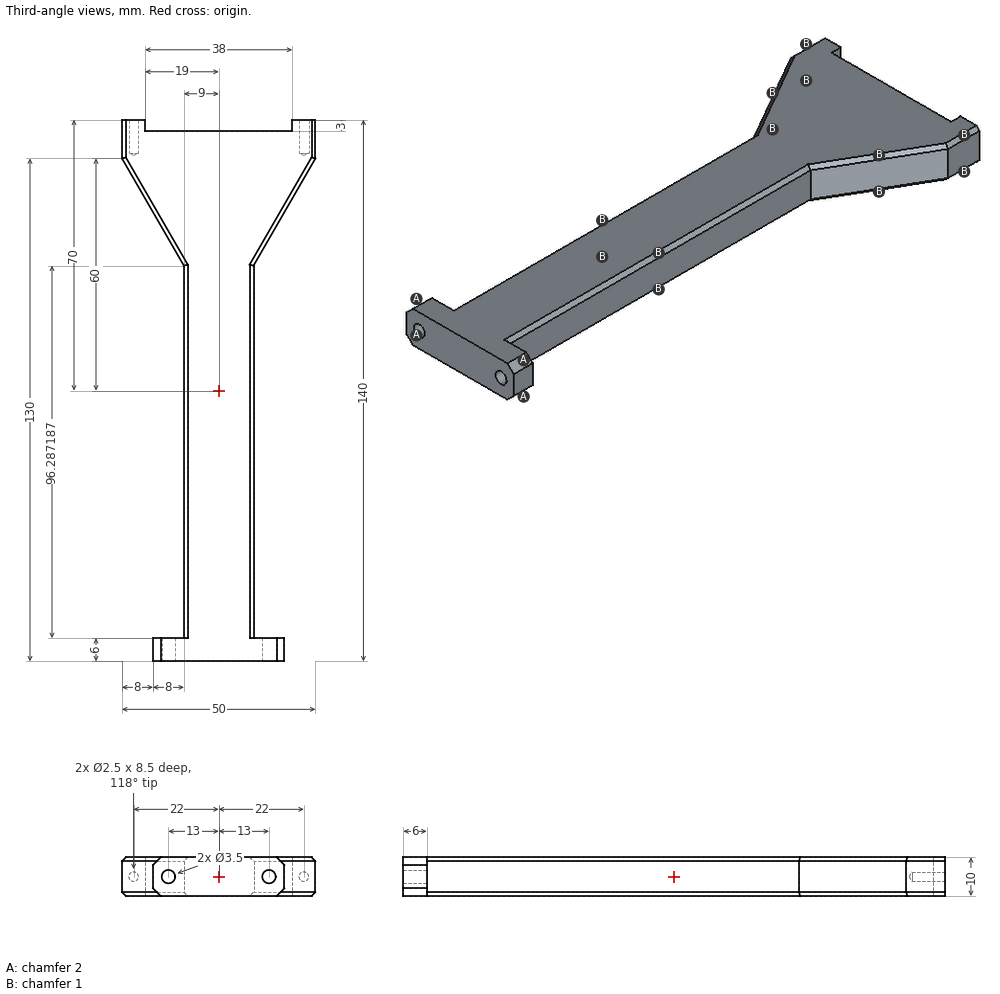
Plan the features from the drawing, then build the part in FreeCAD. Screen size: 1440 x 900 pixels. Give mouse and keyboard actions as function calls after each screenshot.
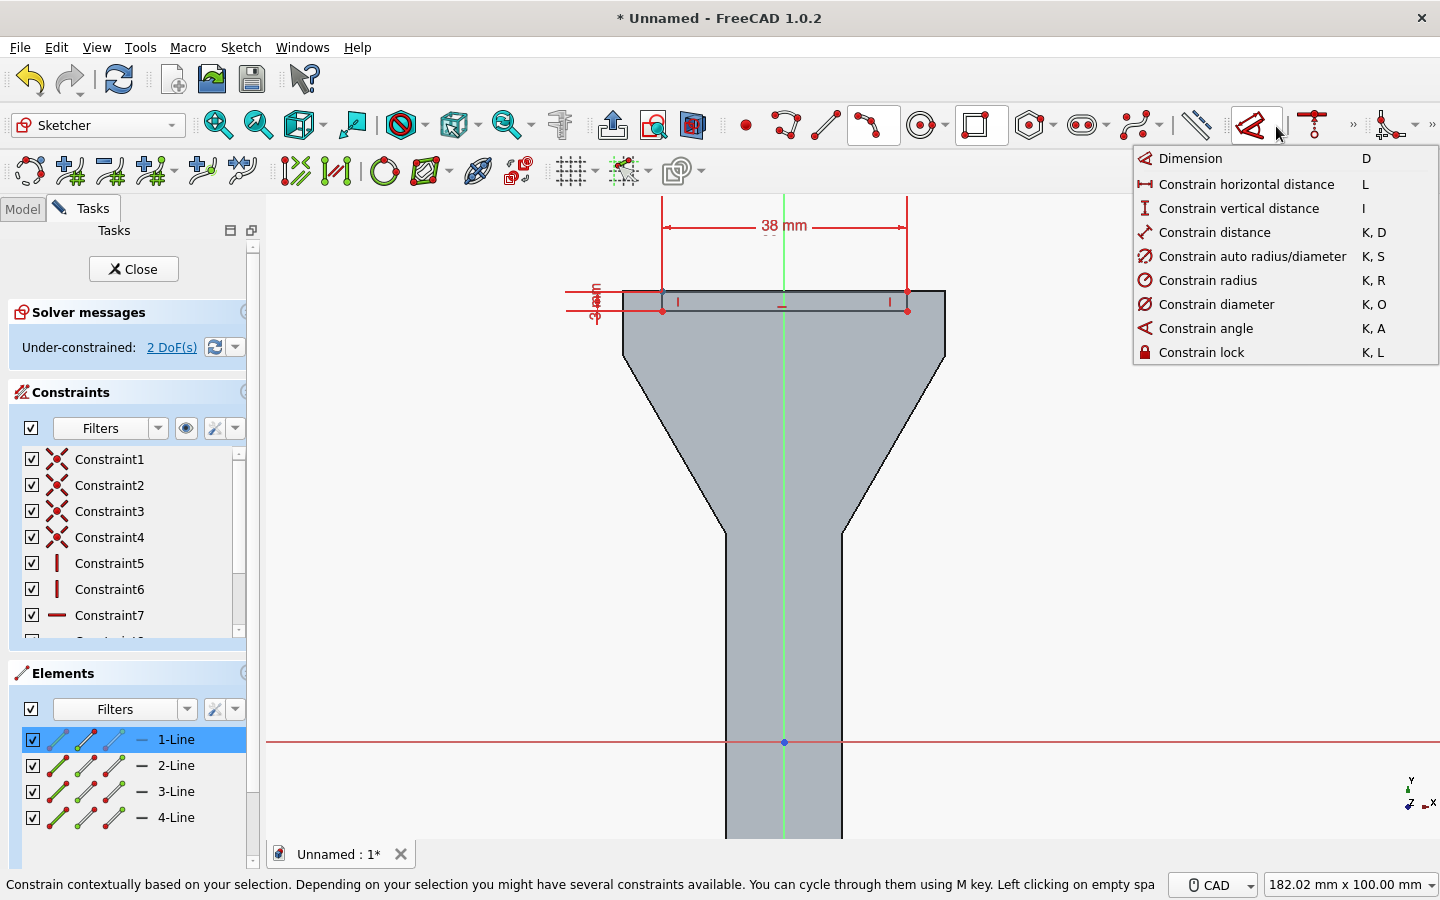
click(1286, 184)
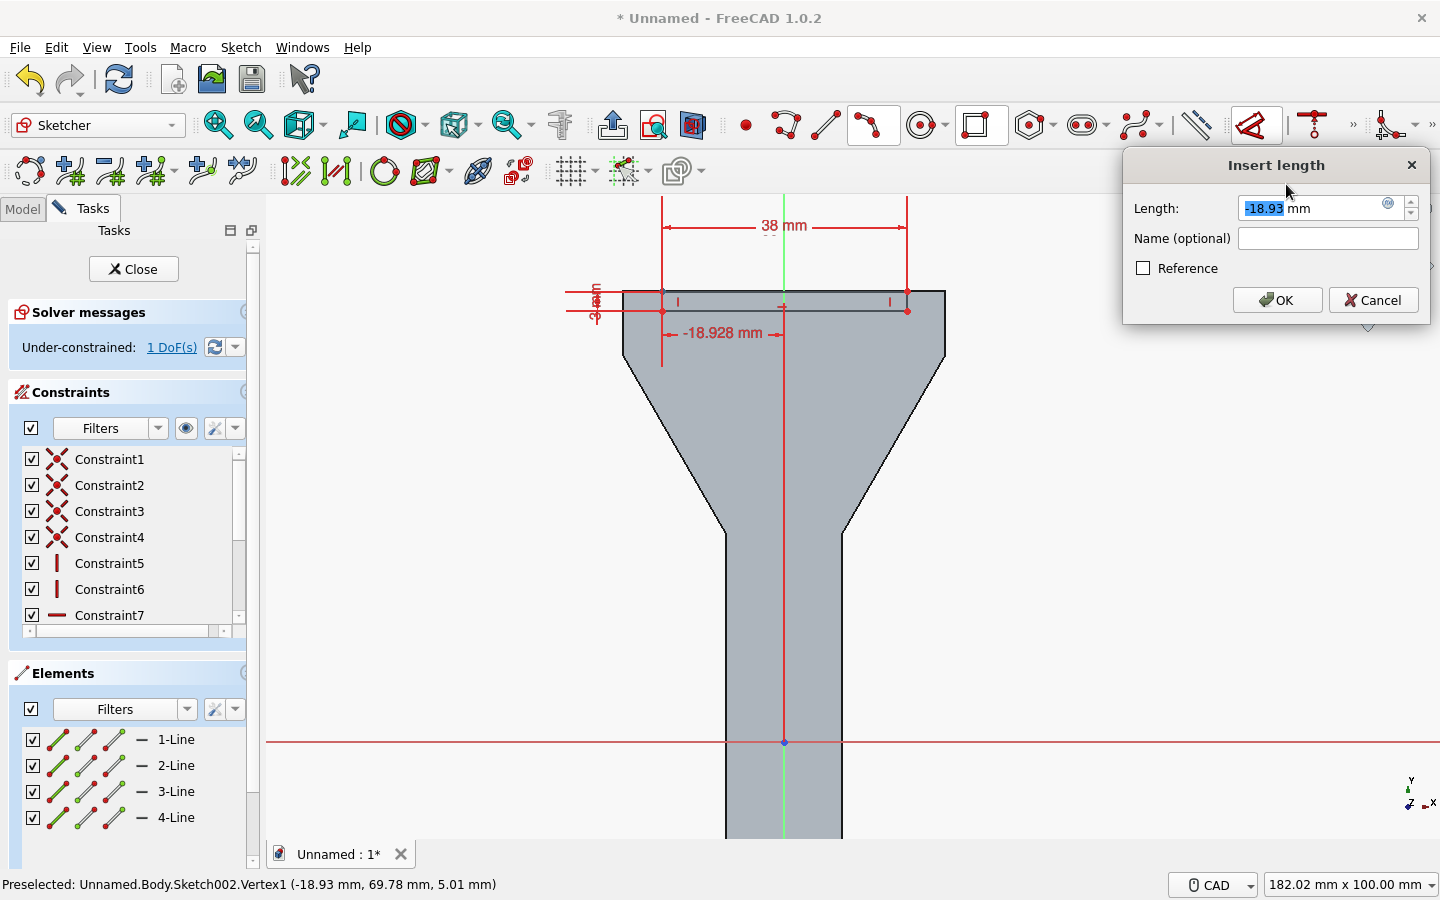
text(-19)
key(Return)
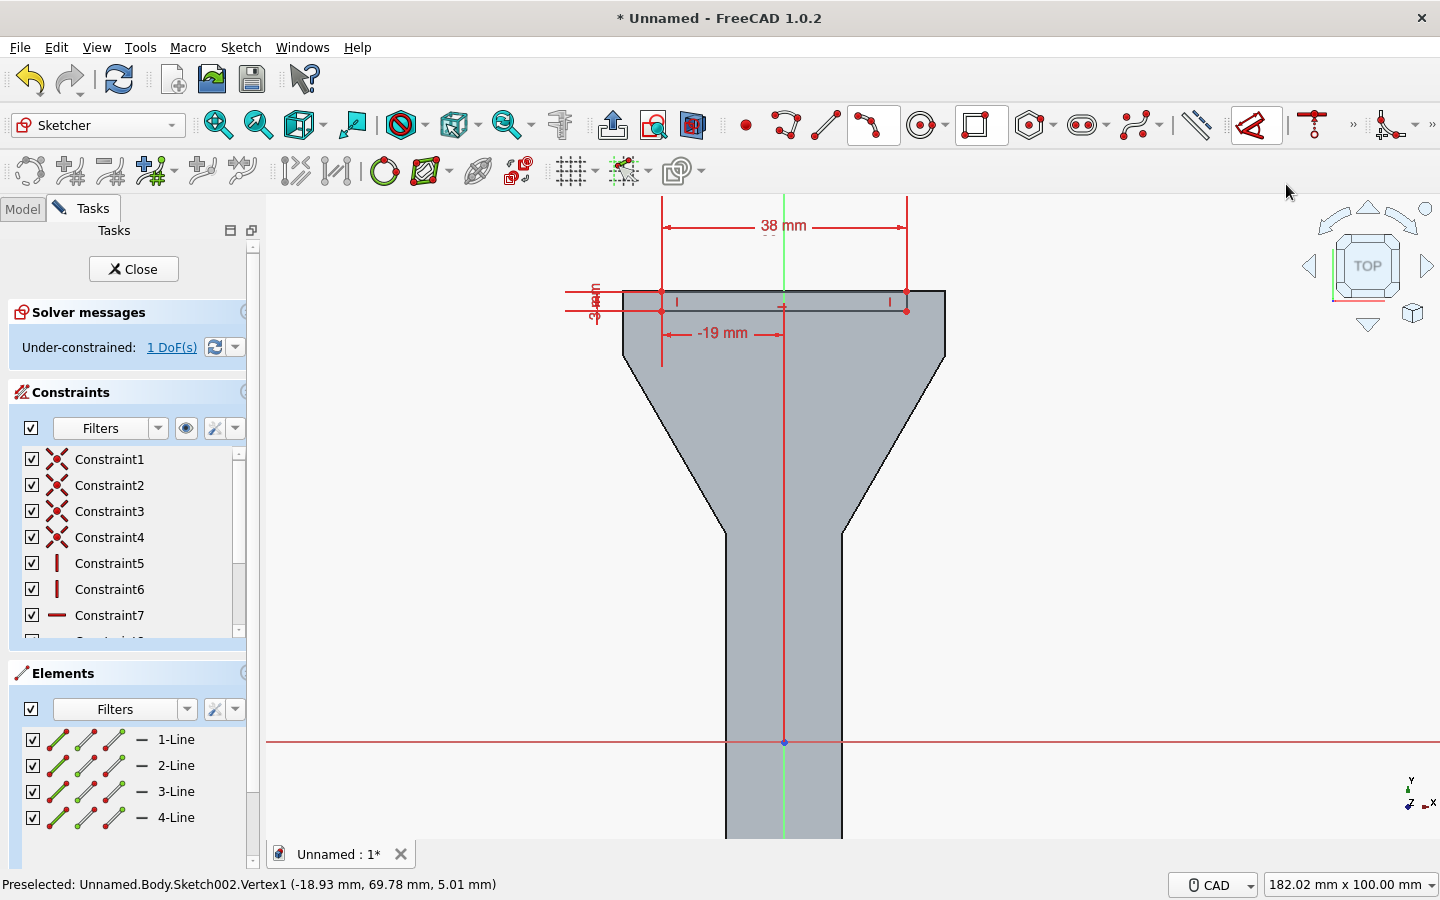
click(662, 292)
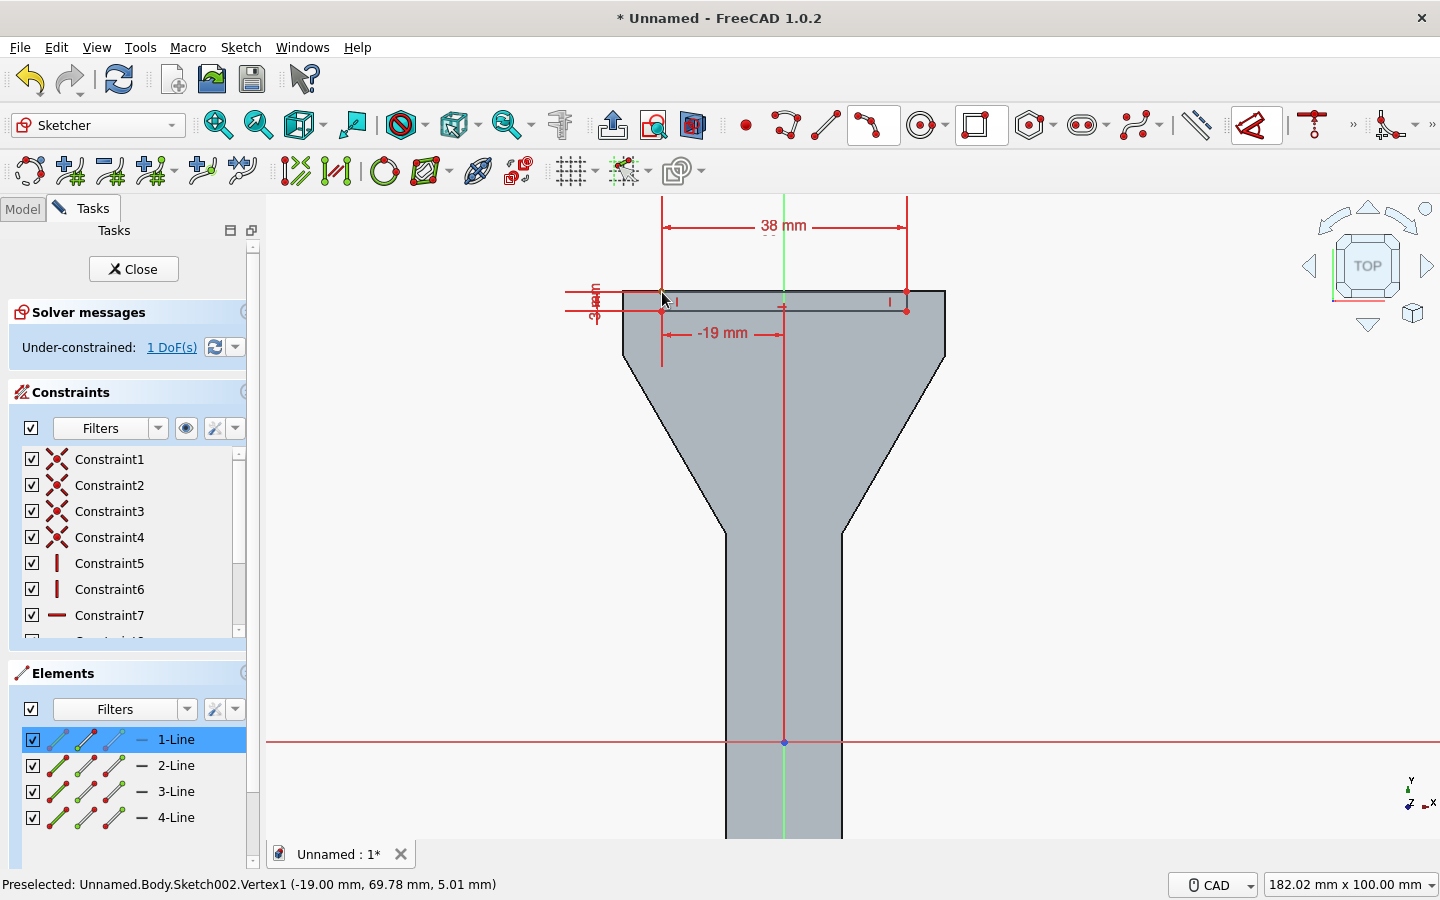
click(1276, 126)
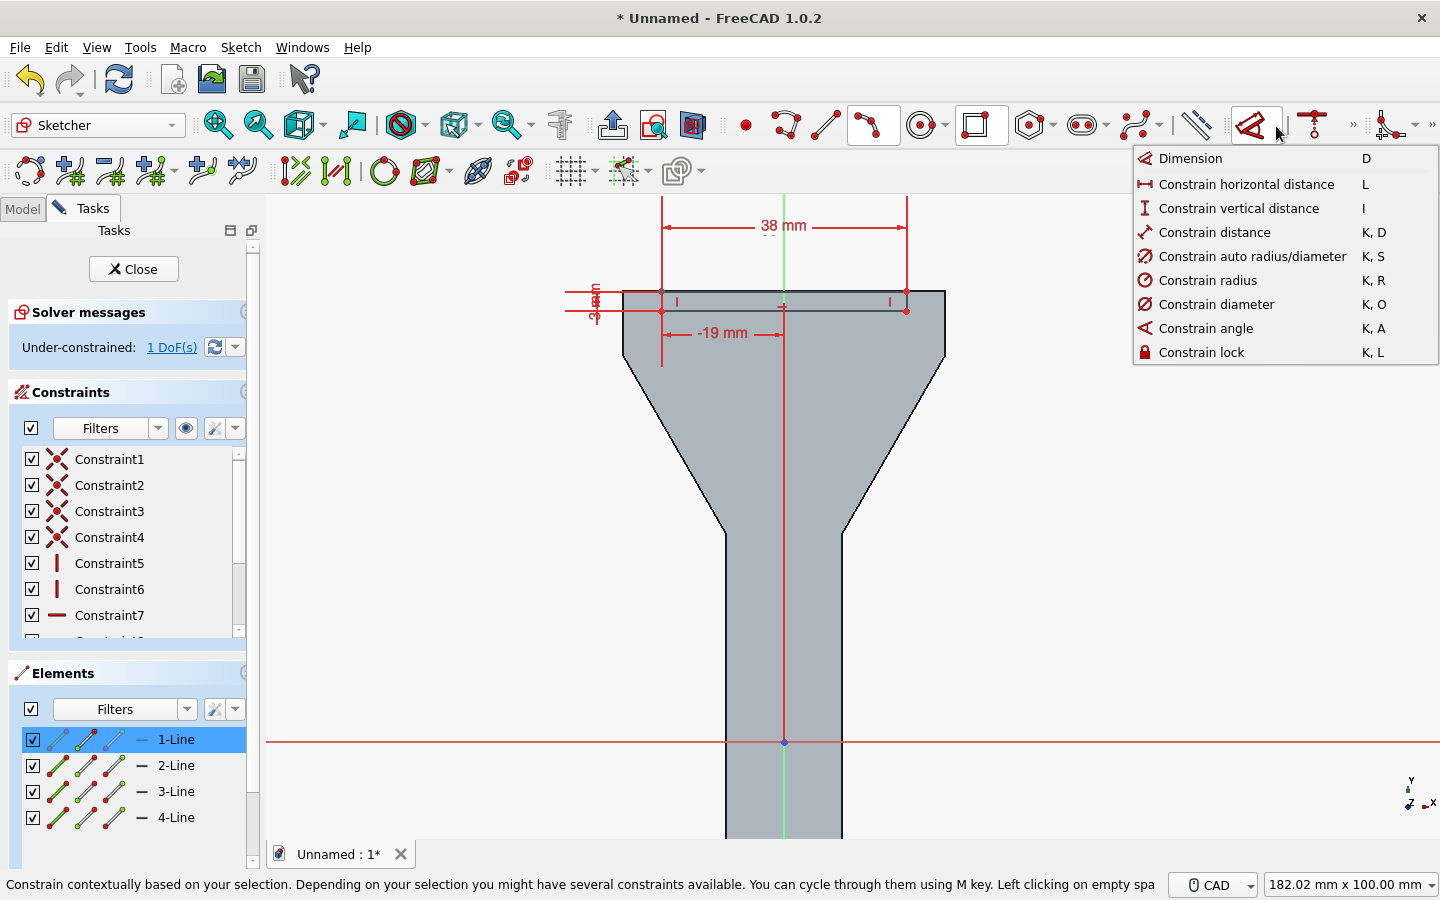
click(1286, 208)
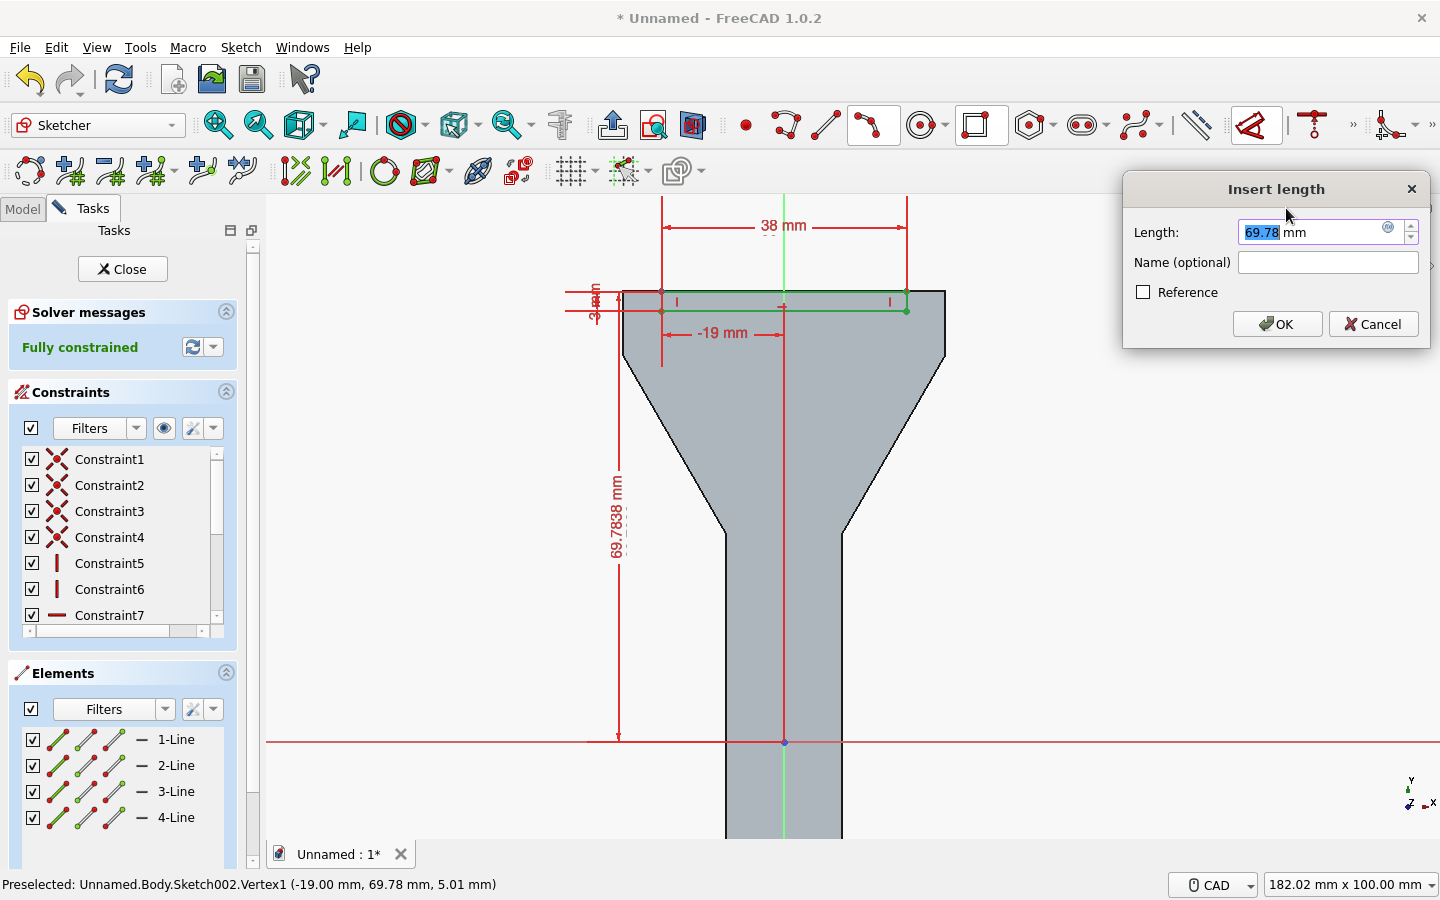
text(70)
key(Return)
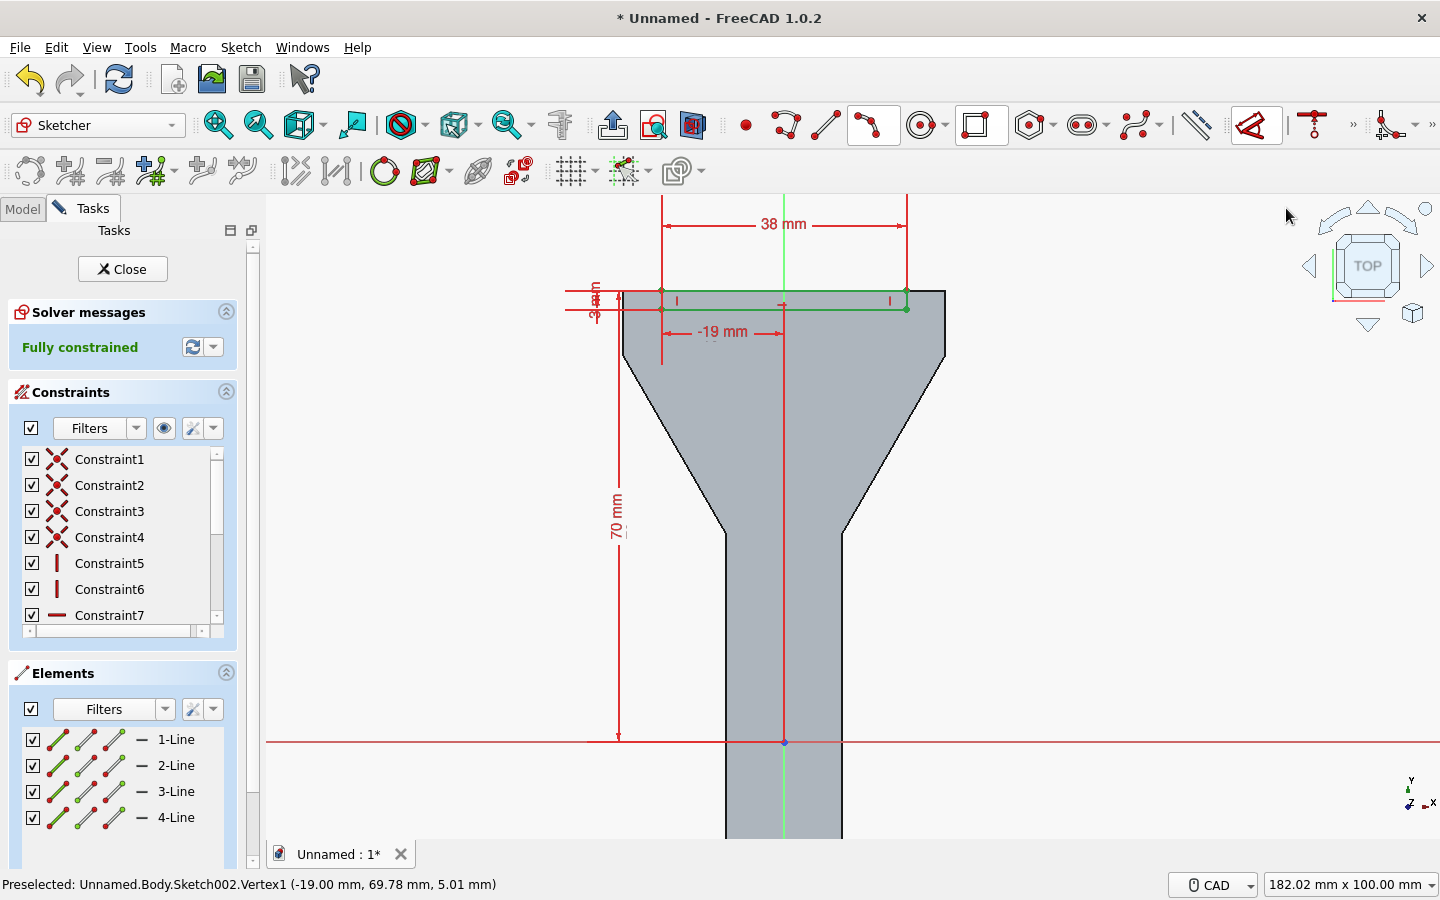
click(123, 269)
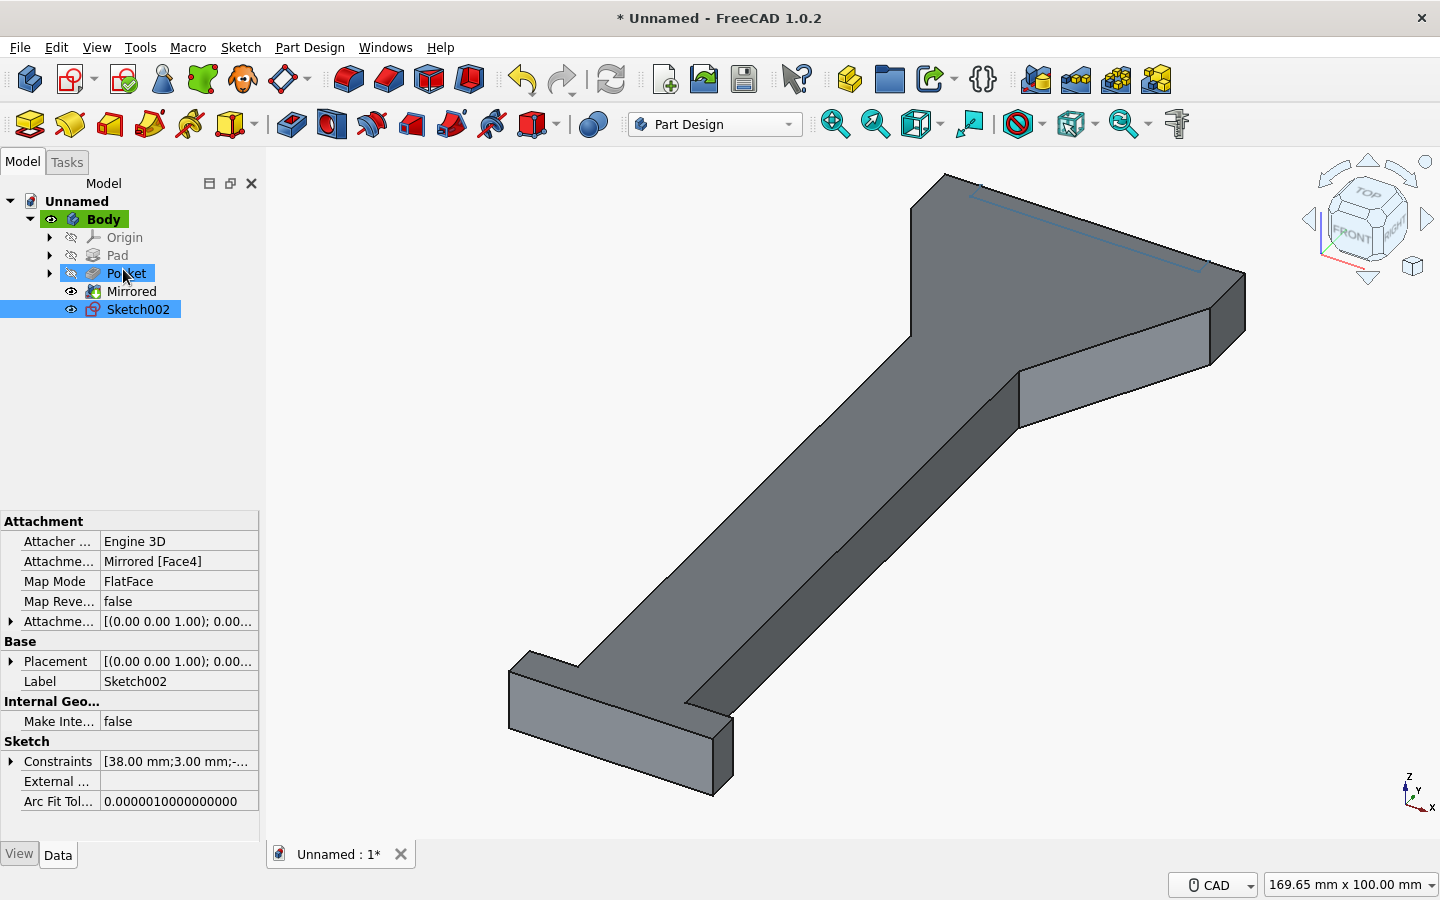
click(292, 124)